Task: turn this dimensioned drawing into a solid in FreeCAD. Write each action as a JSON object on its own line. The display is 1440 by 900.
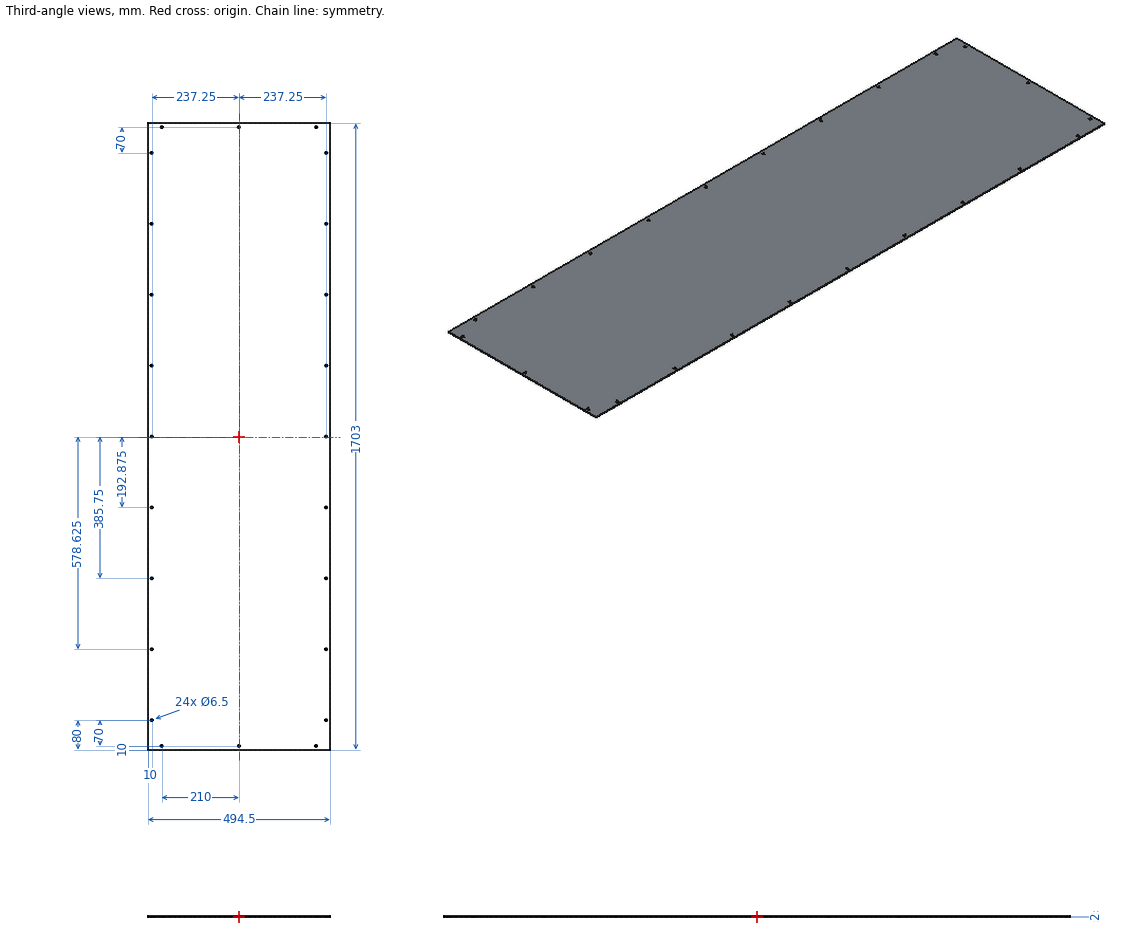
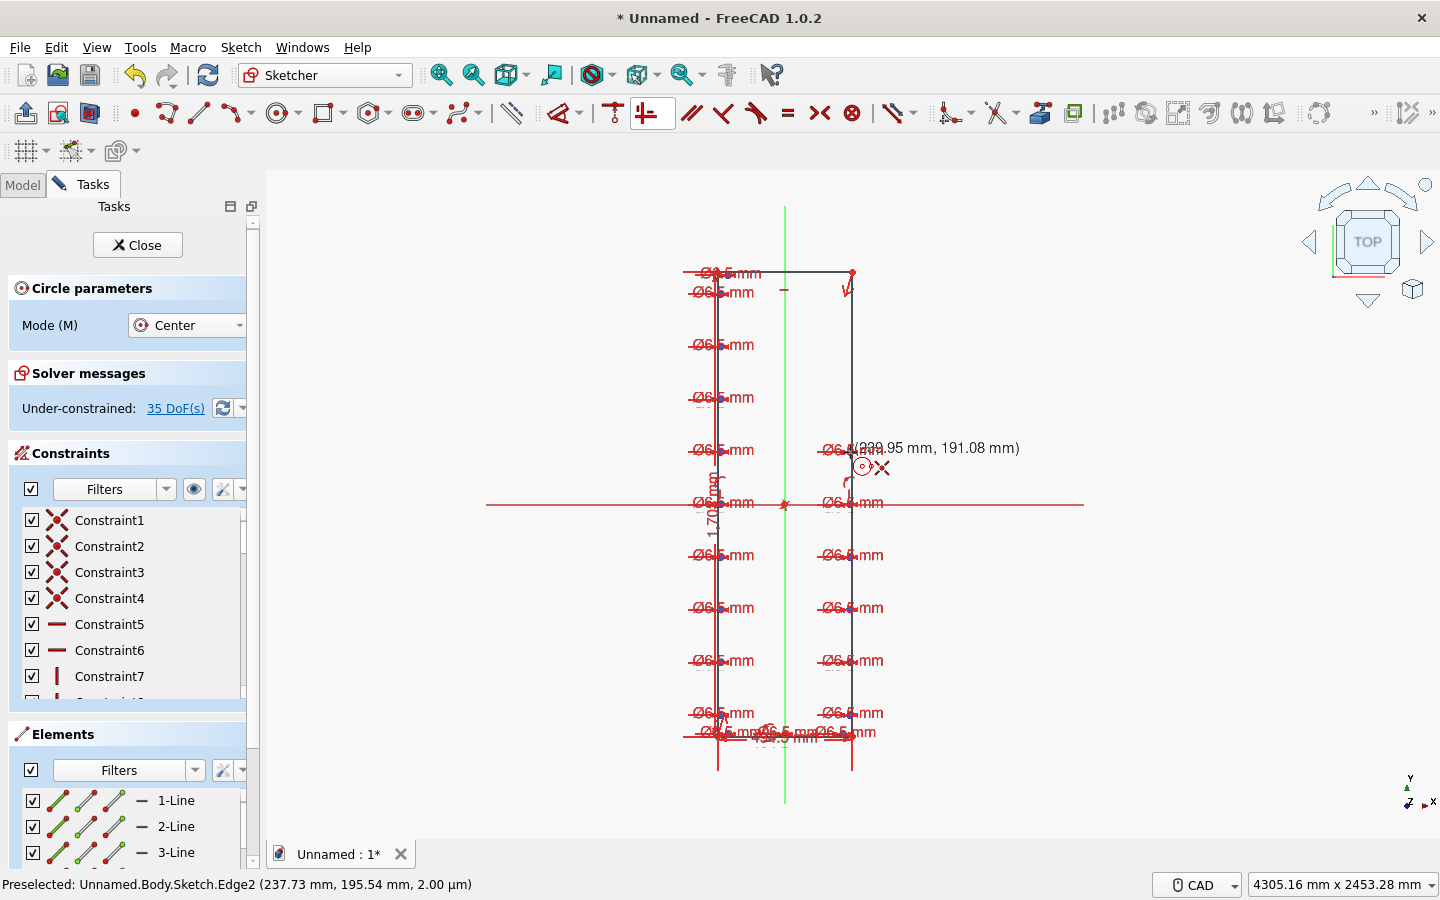
{"action": "scroll", "coordinate": [850, 399], "scroll_direction": "up", "scroll_amount": 17}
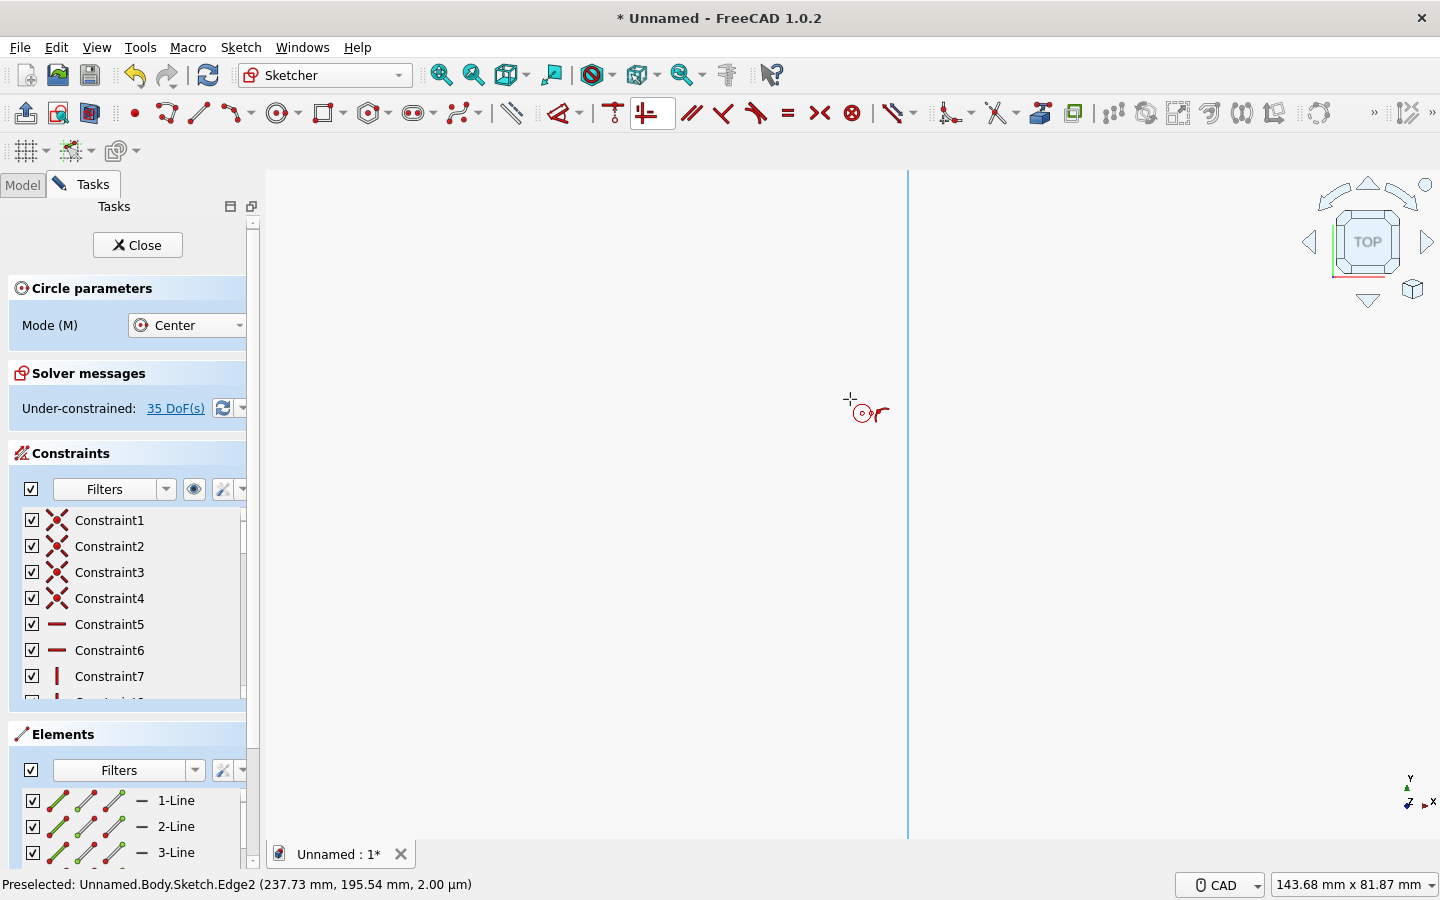
{"action": "scroll", "coordinate": [850, 399], "scroll_direction": "down", "scroll_amount": 17}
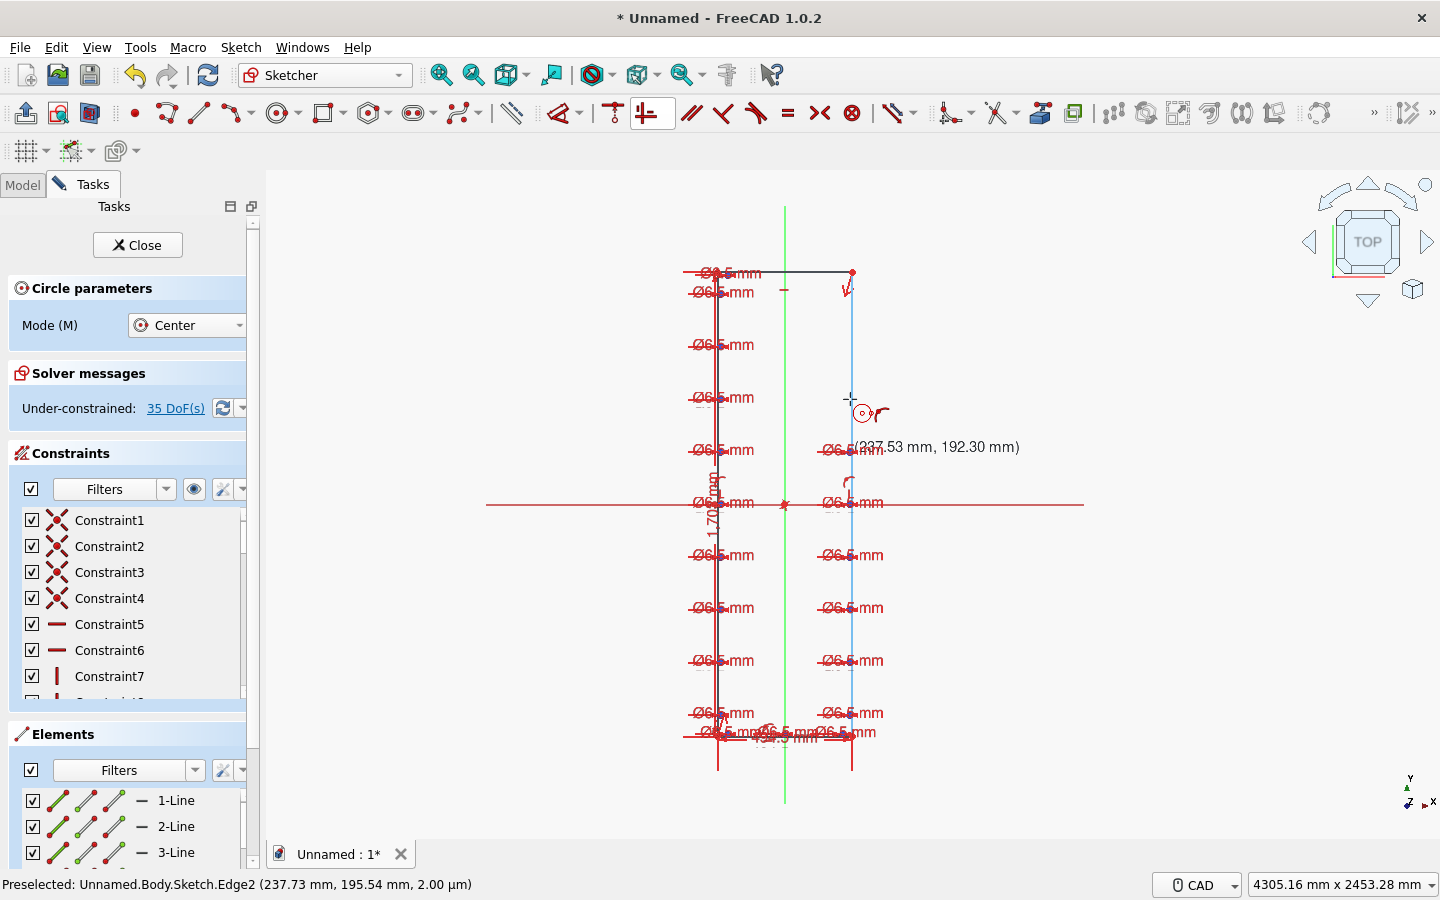
{"action": "scroll", "coordinate": [850, 399], "scroll_direction": "up", "scroll_amount": 9}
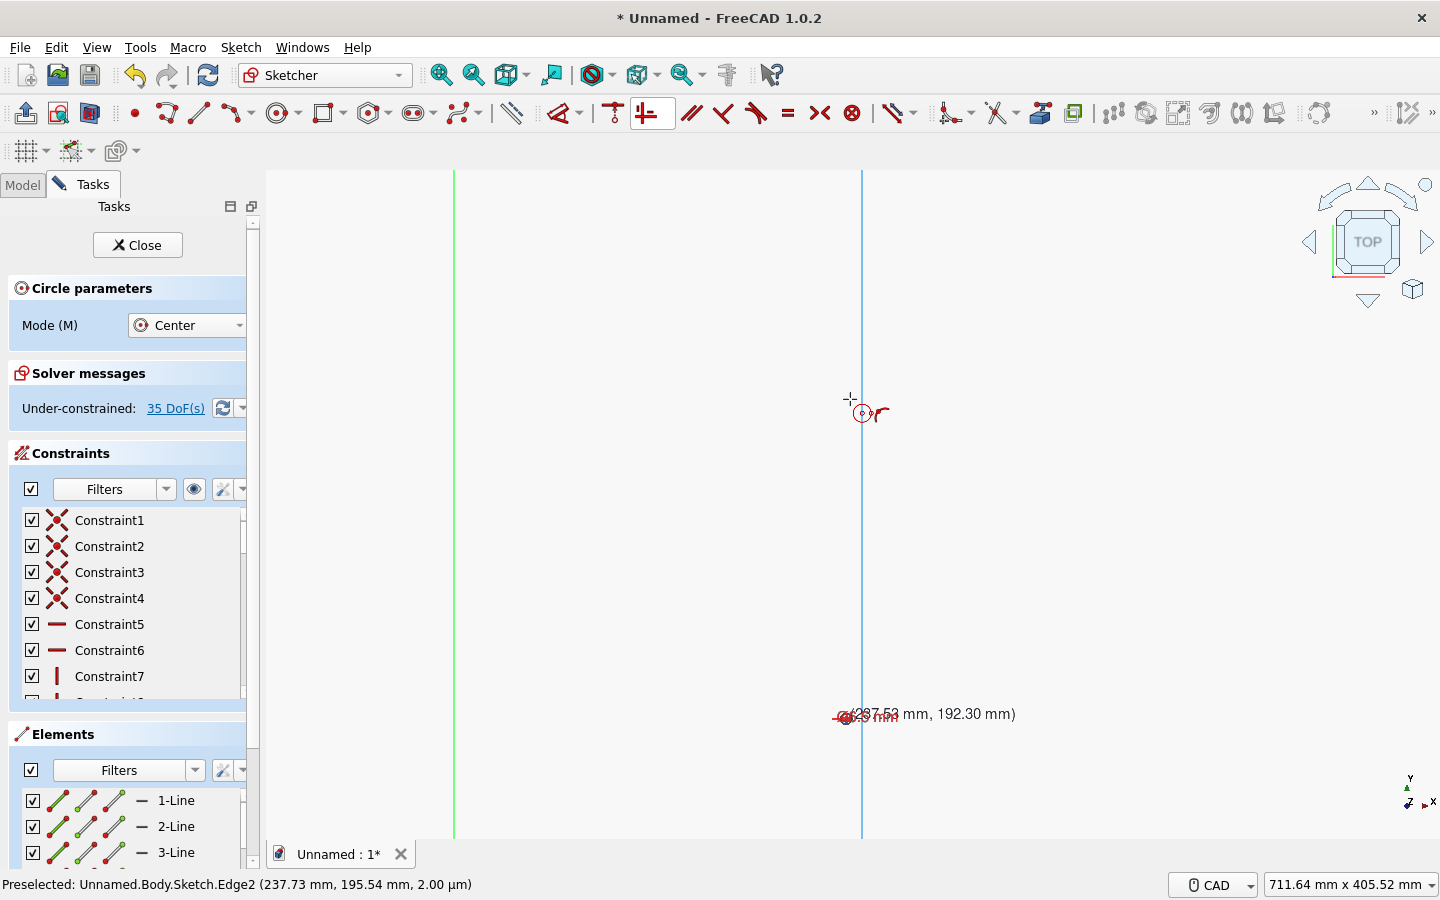
{"action": "left_click", "coordinate": [846, 400]}
{"action": "mouse_move", "coordinate": [842, 396]}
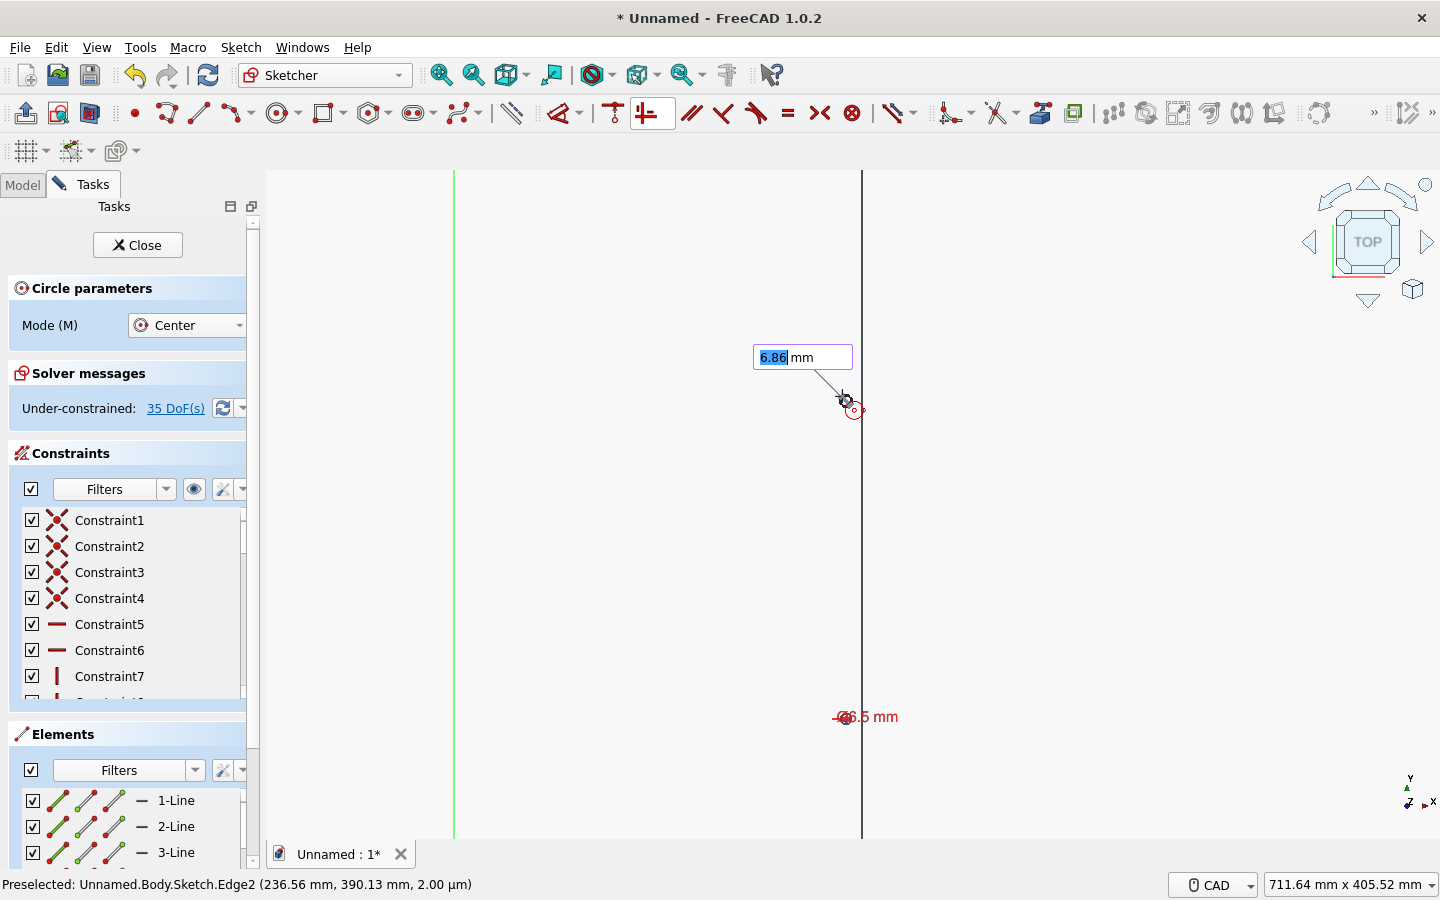
{"action": "type", "text": "6.5"}
{"action": "key", "text": "Return"}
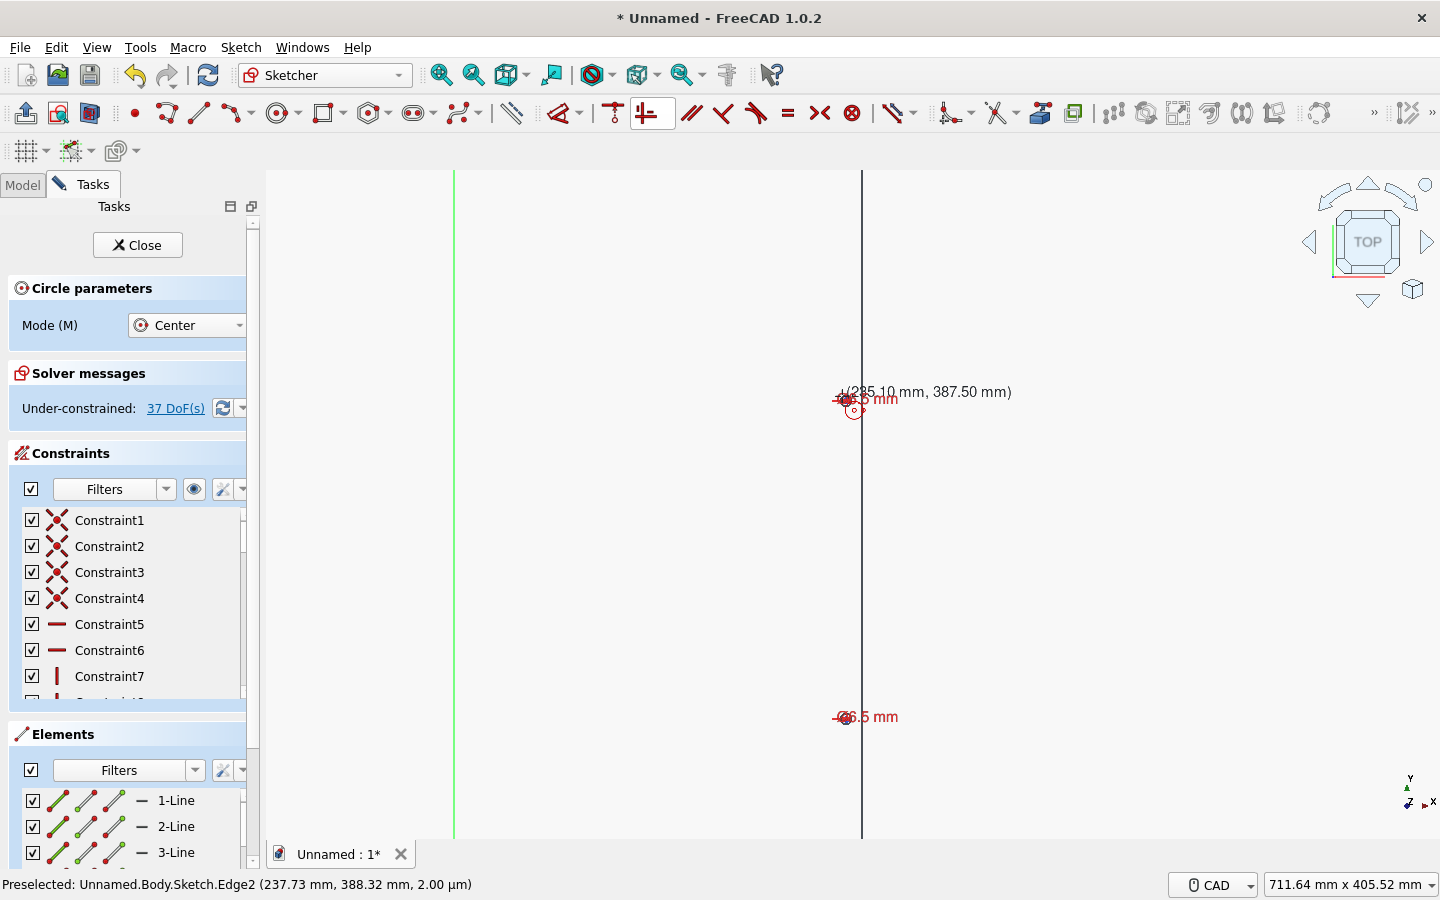
{"action": "scroll", "coordinate": [850, 399], "scroll_direction": "down", "scroll_amount": 9}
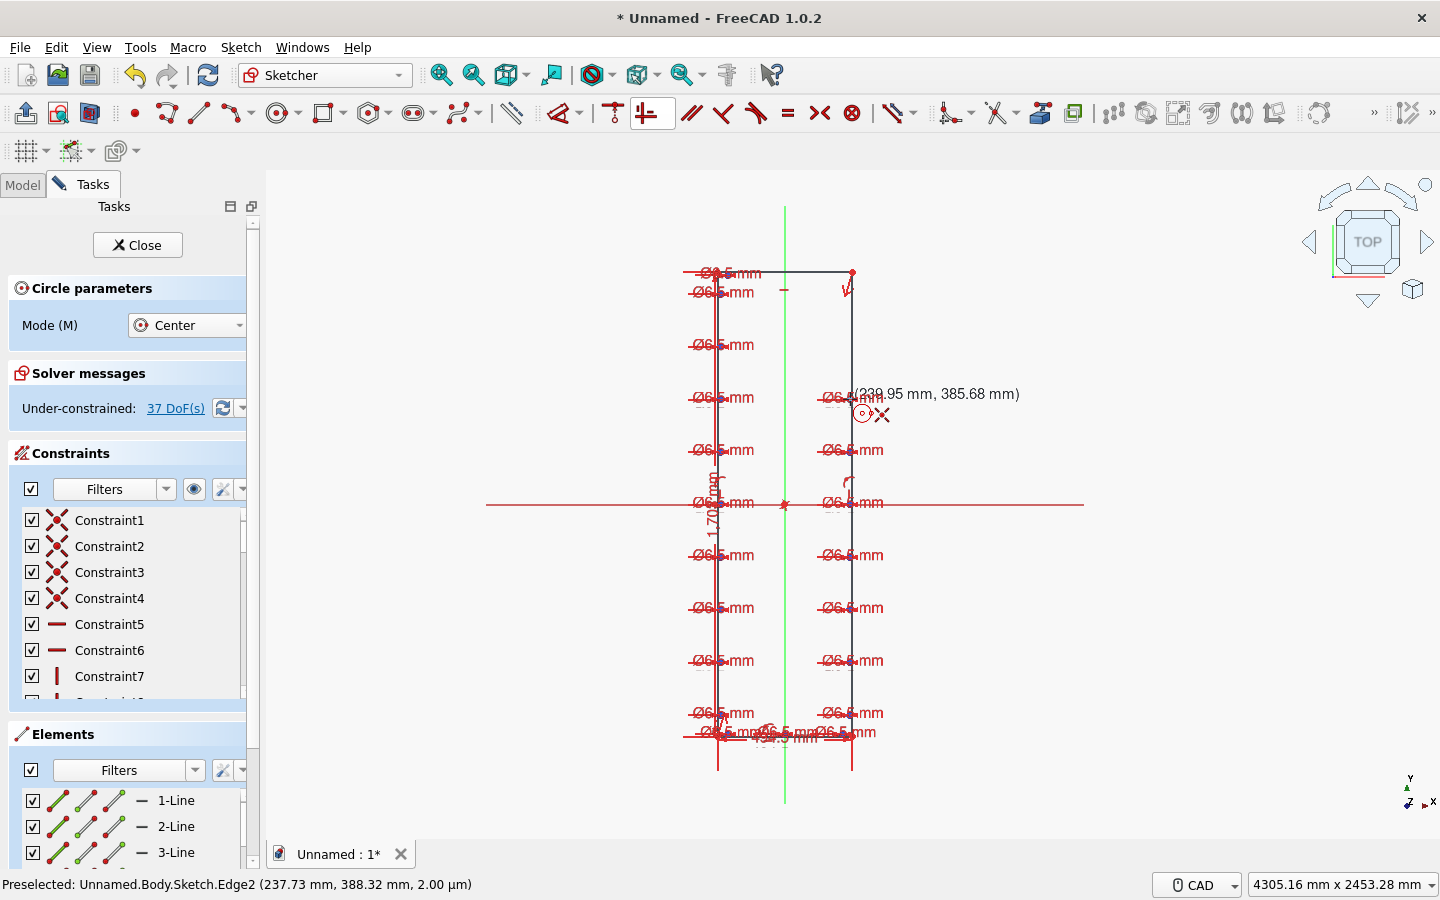
{"action": "scroll", "coordinate": [785, 275], "scroll_direction": "up", "scroll_amount": 17}